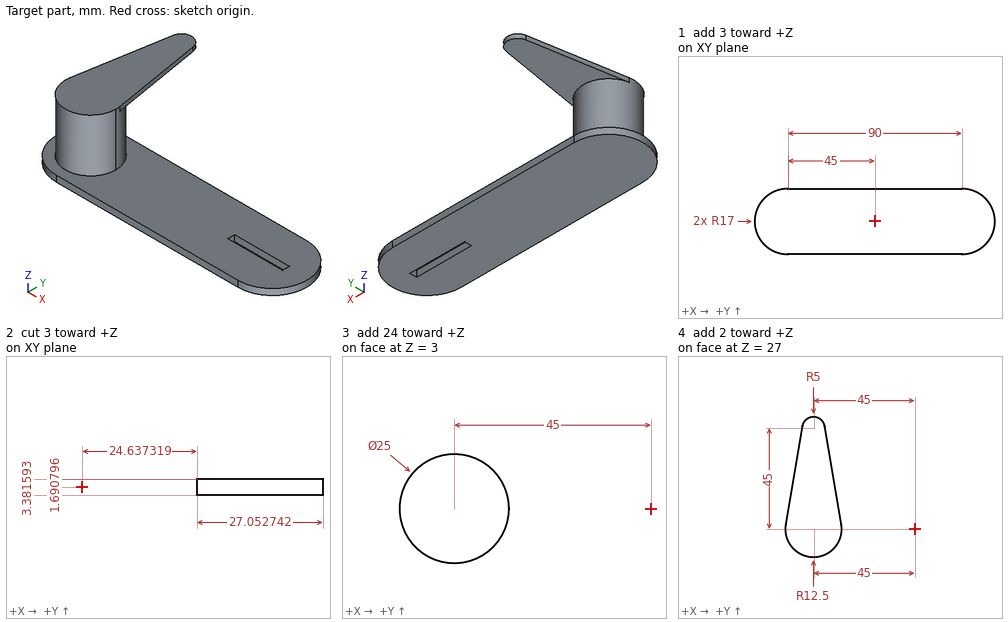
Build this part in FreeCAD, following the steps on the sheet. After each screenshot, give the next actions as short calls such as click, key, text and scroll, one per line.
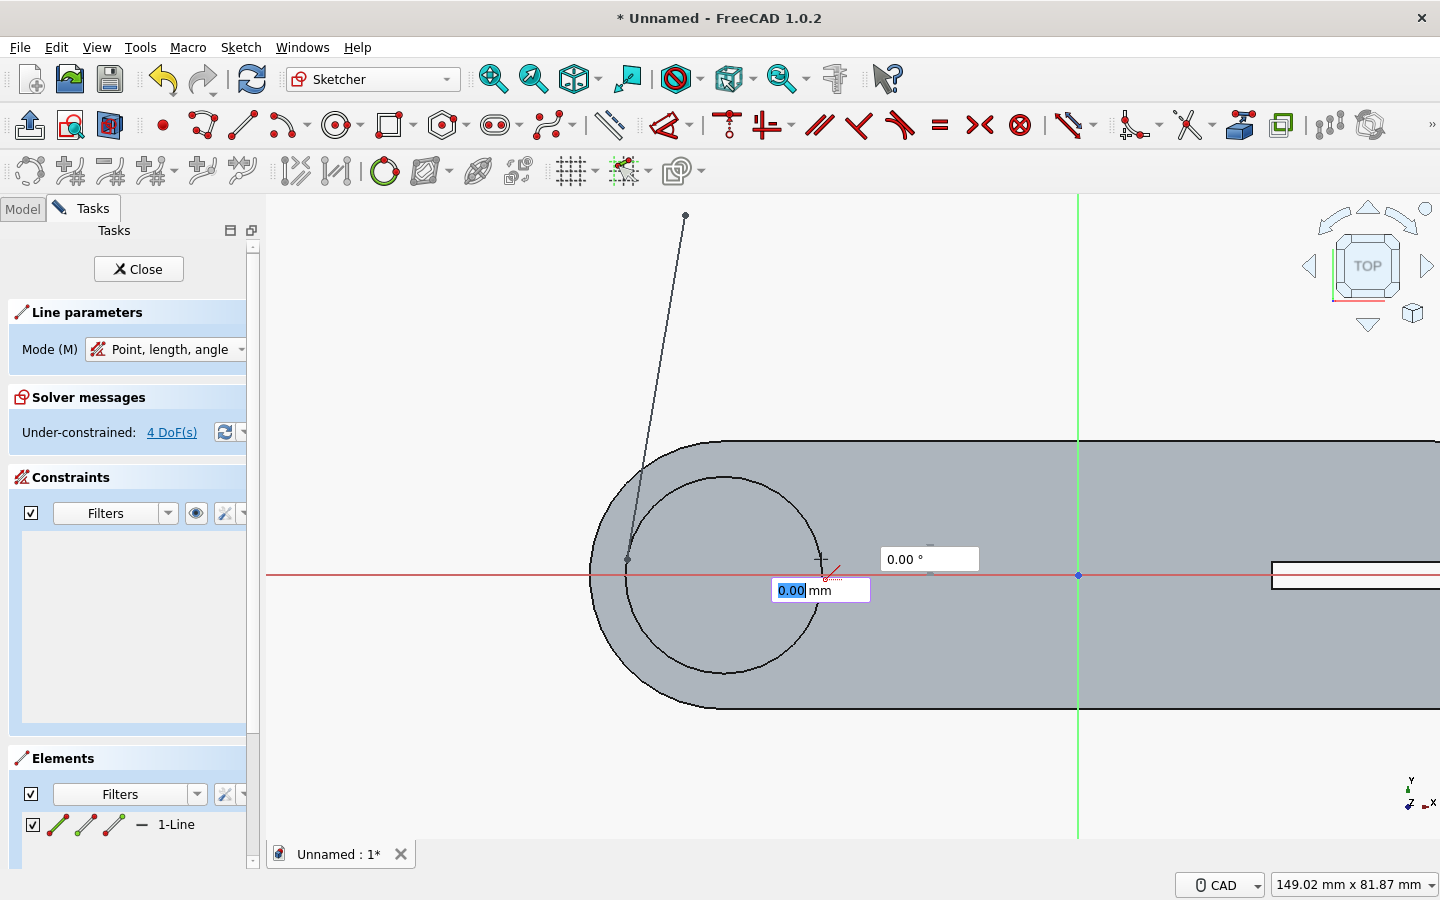
scroll(477, 811, down, 1)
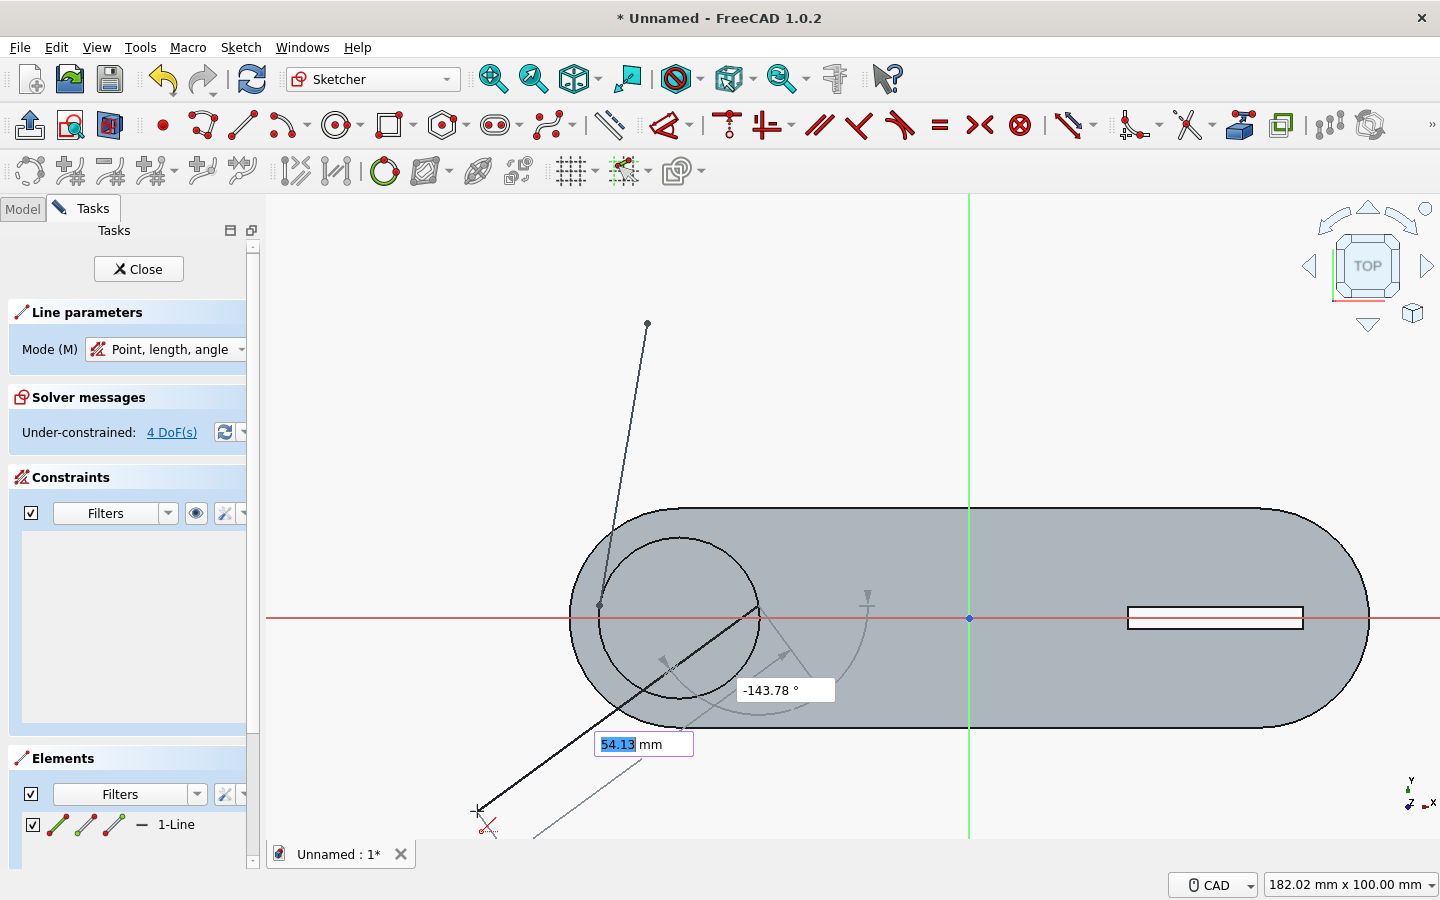
click(711, 323)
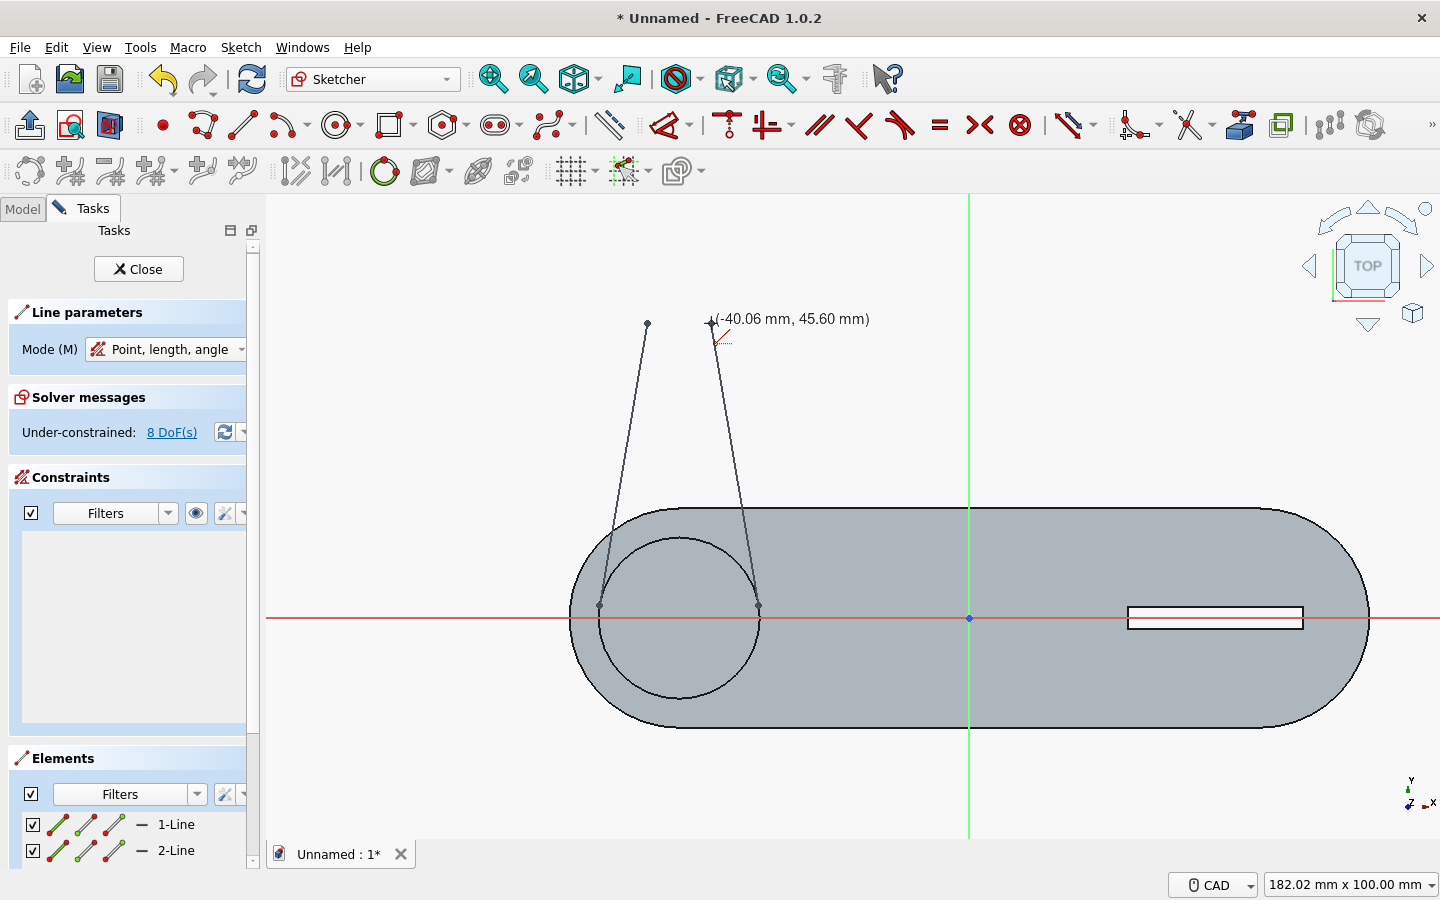
click(310, 126)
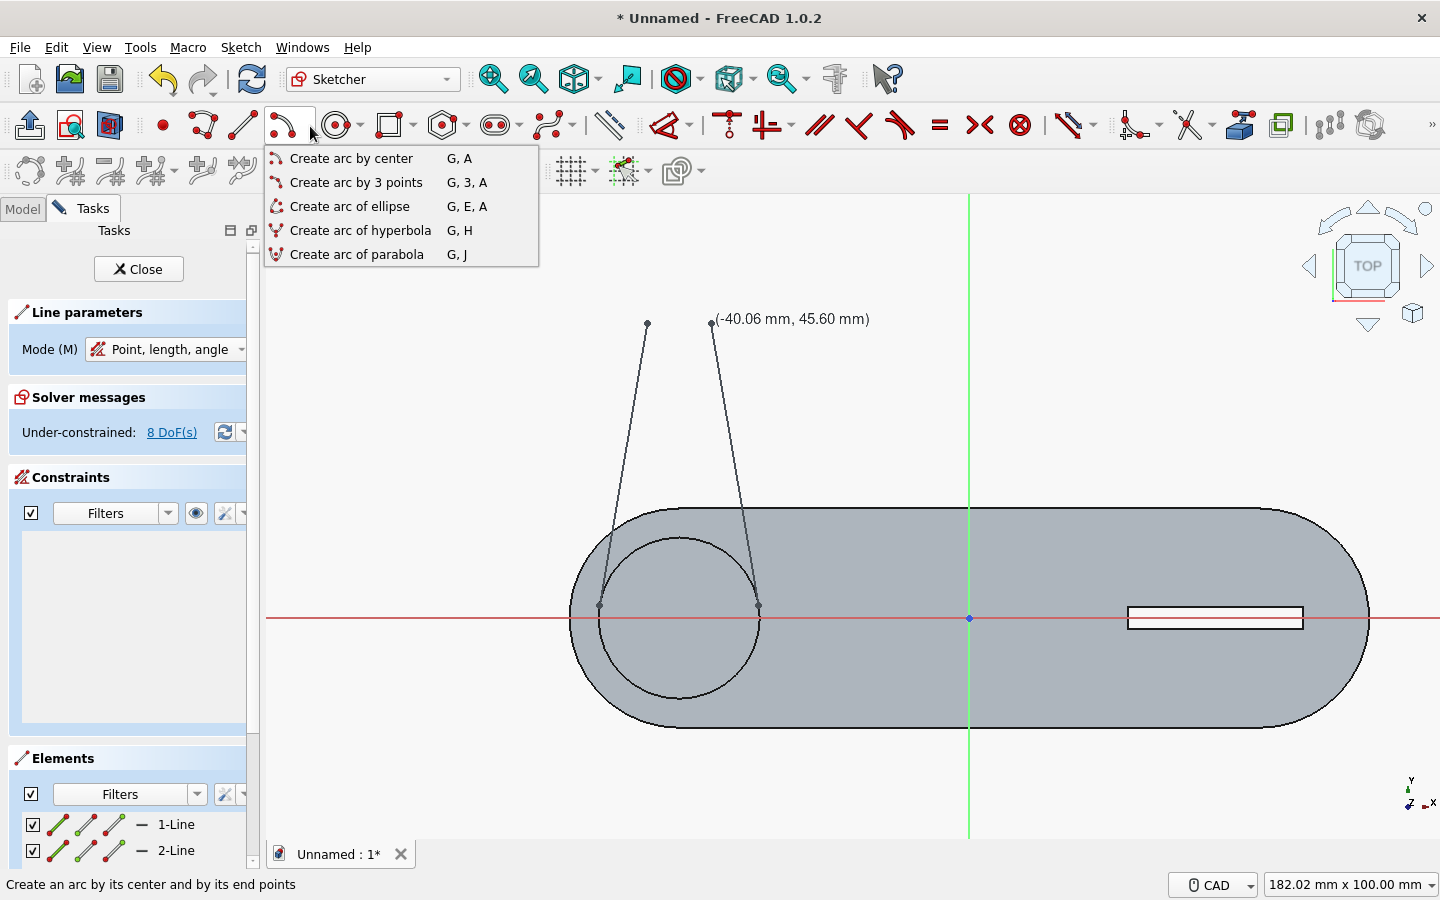
click(402, 182)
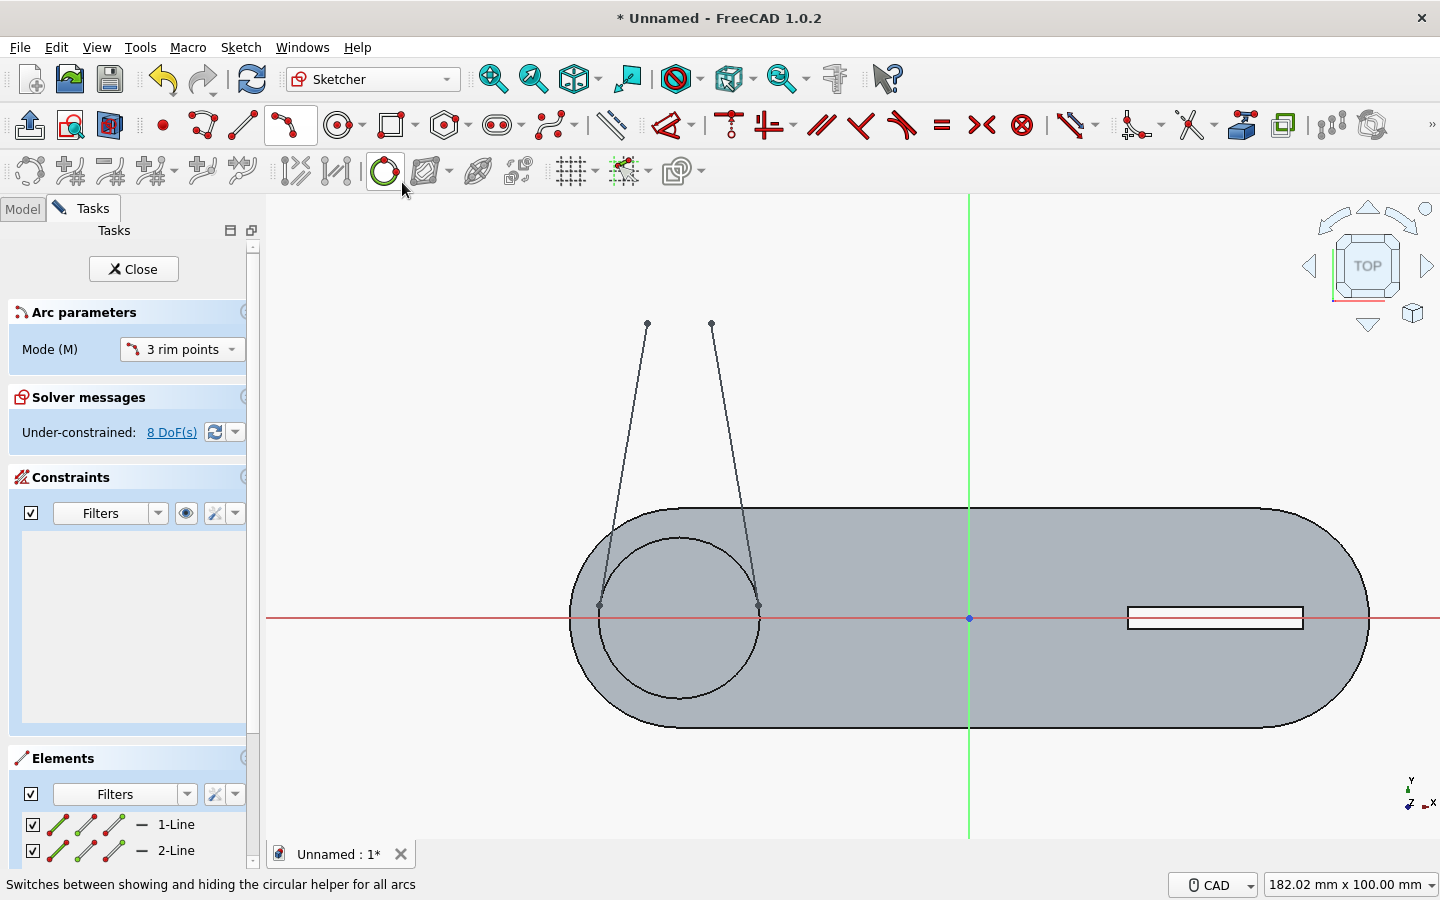
click(600, 606)
click(759, 606)
click(679, 699)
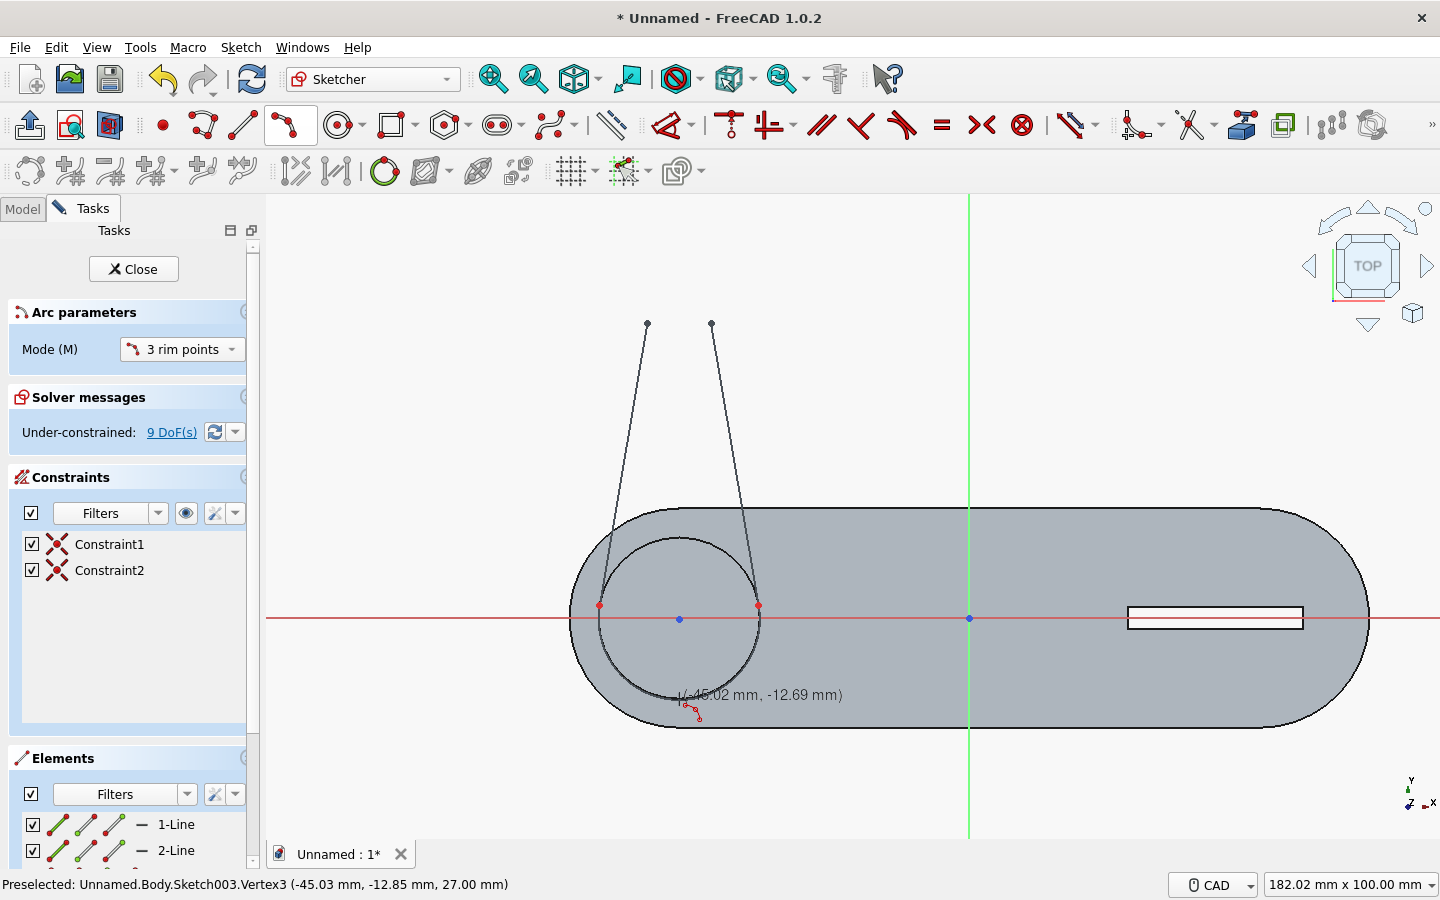
click(711, 324)
click(647, 324)
click(679, 296)
key(Escape)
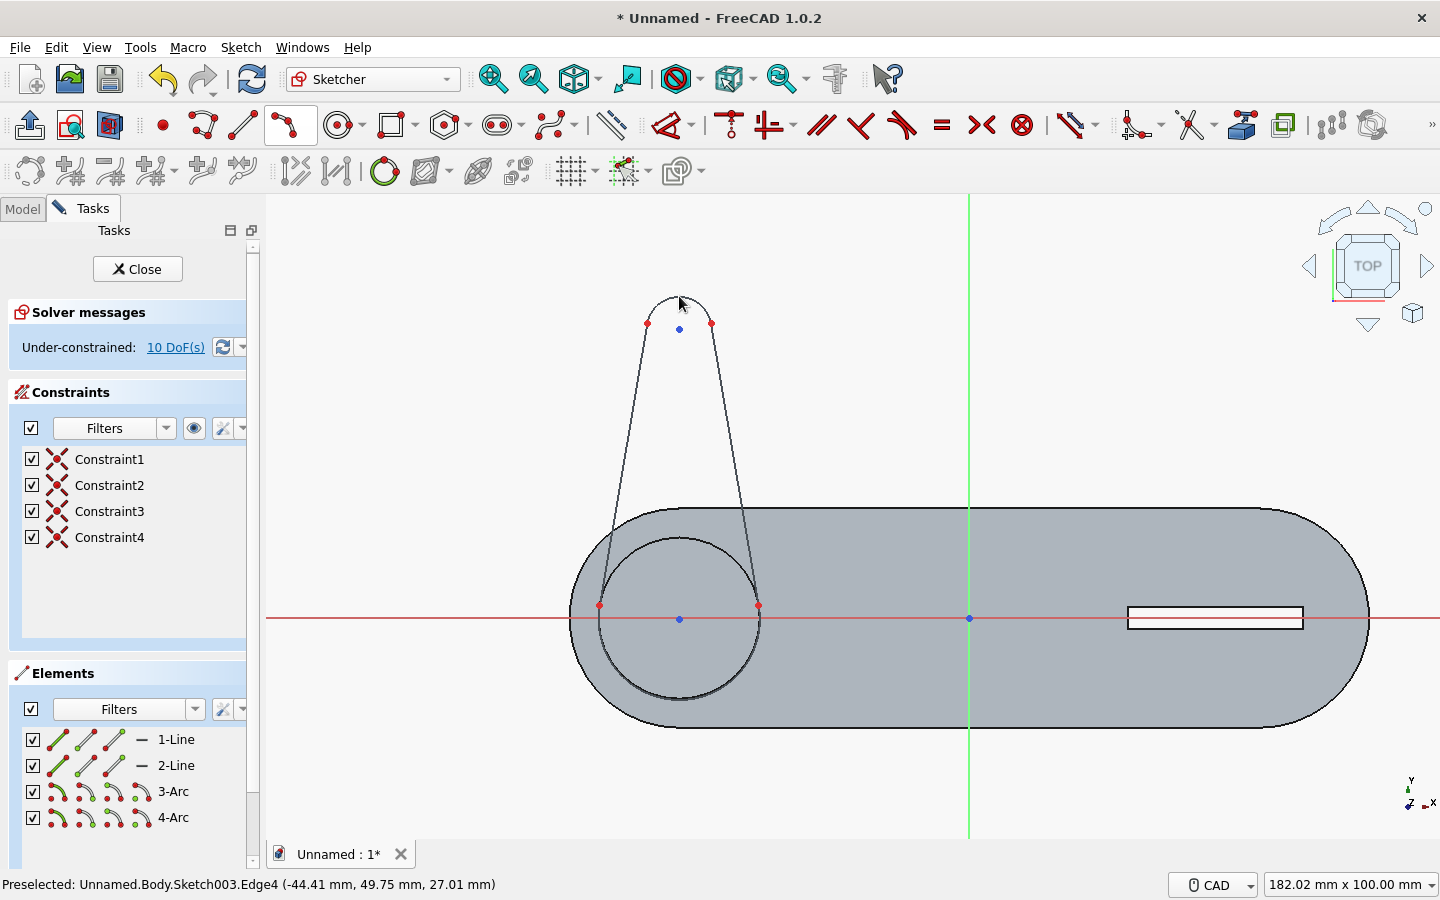
click(633, 408)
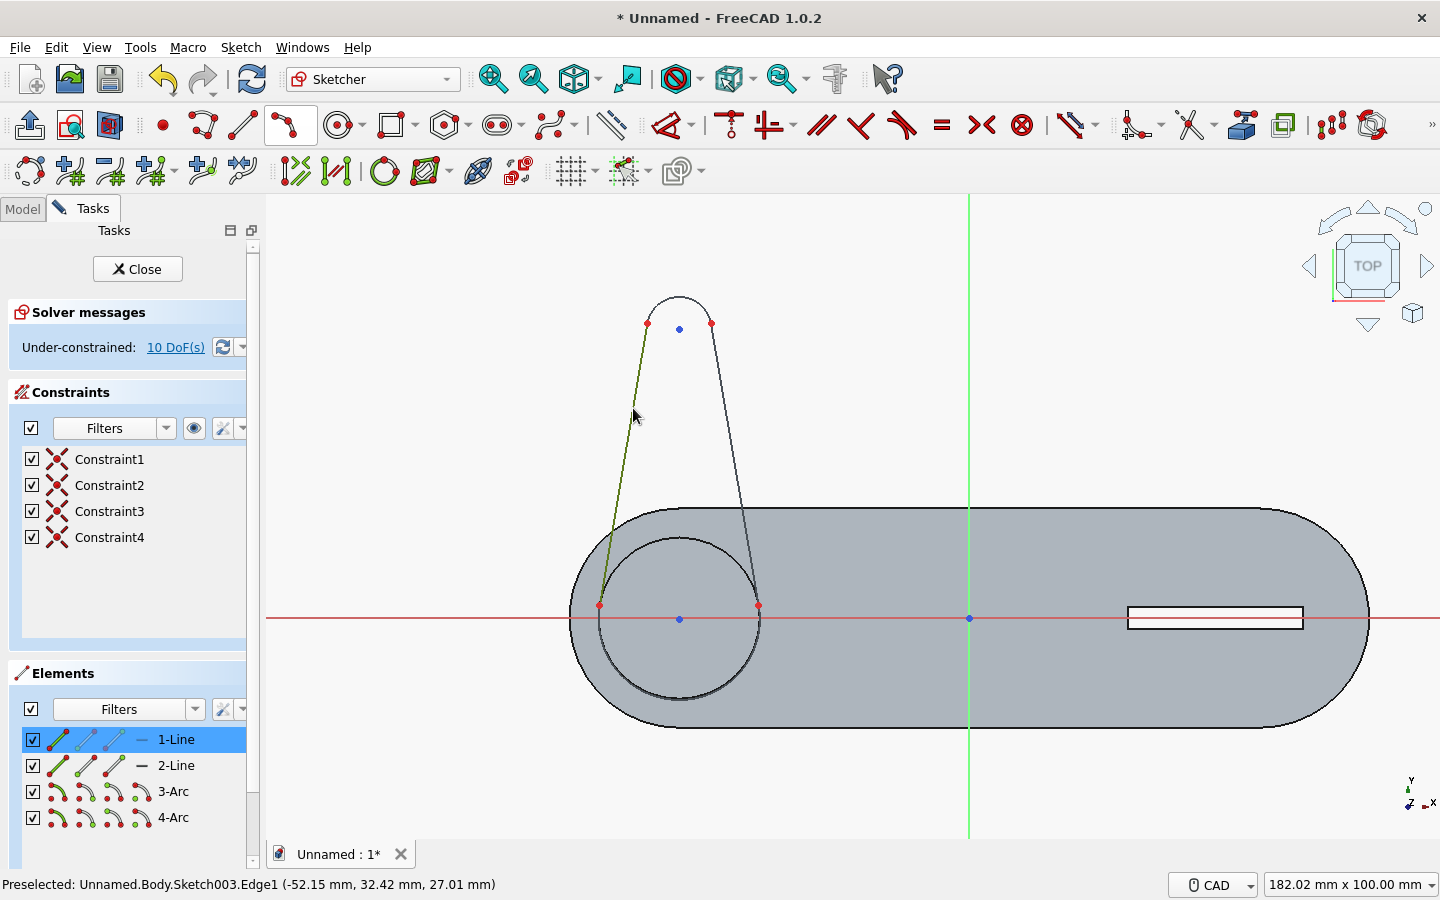
click(628, 681)